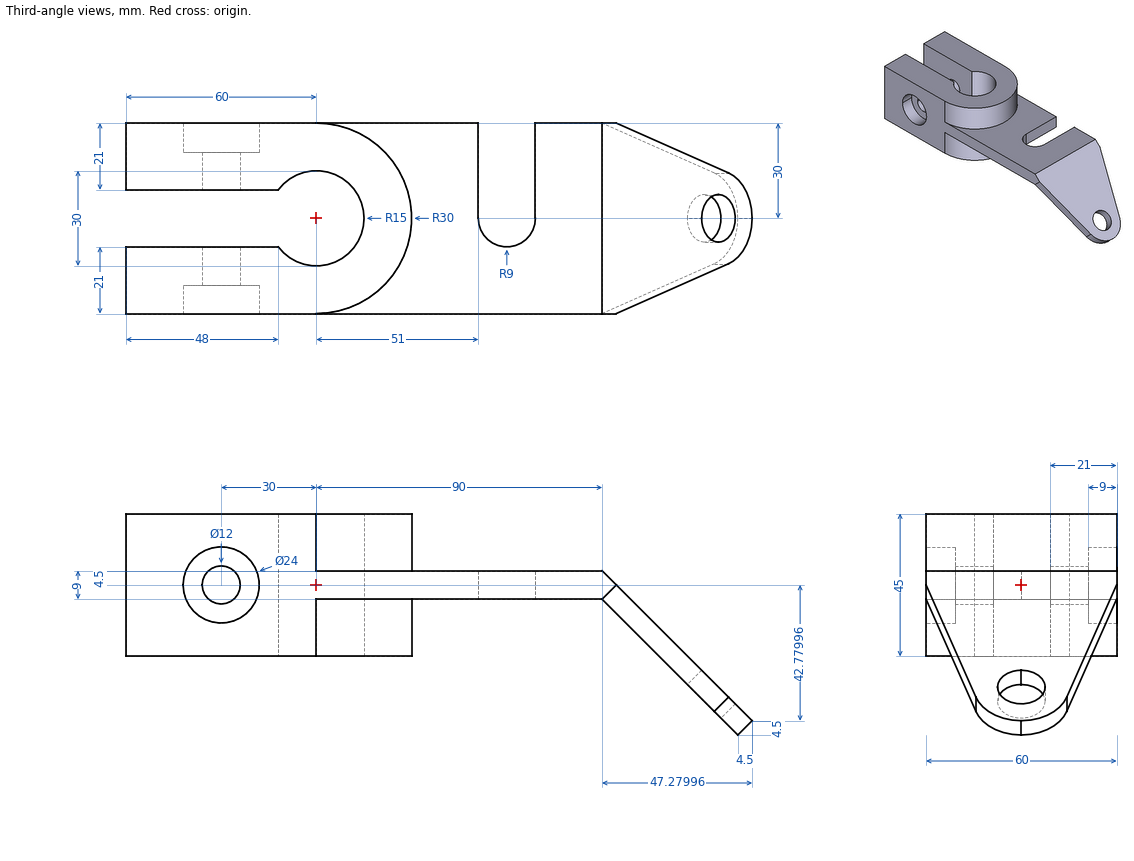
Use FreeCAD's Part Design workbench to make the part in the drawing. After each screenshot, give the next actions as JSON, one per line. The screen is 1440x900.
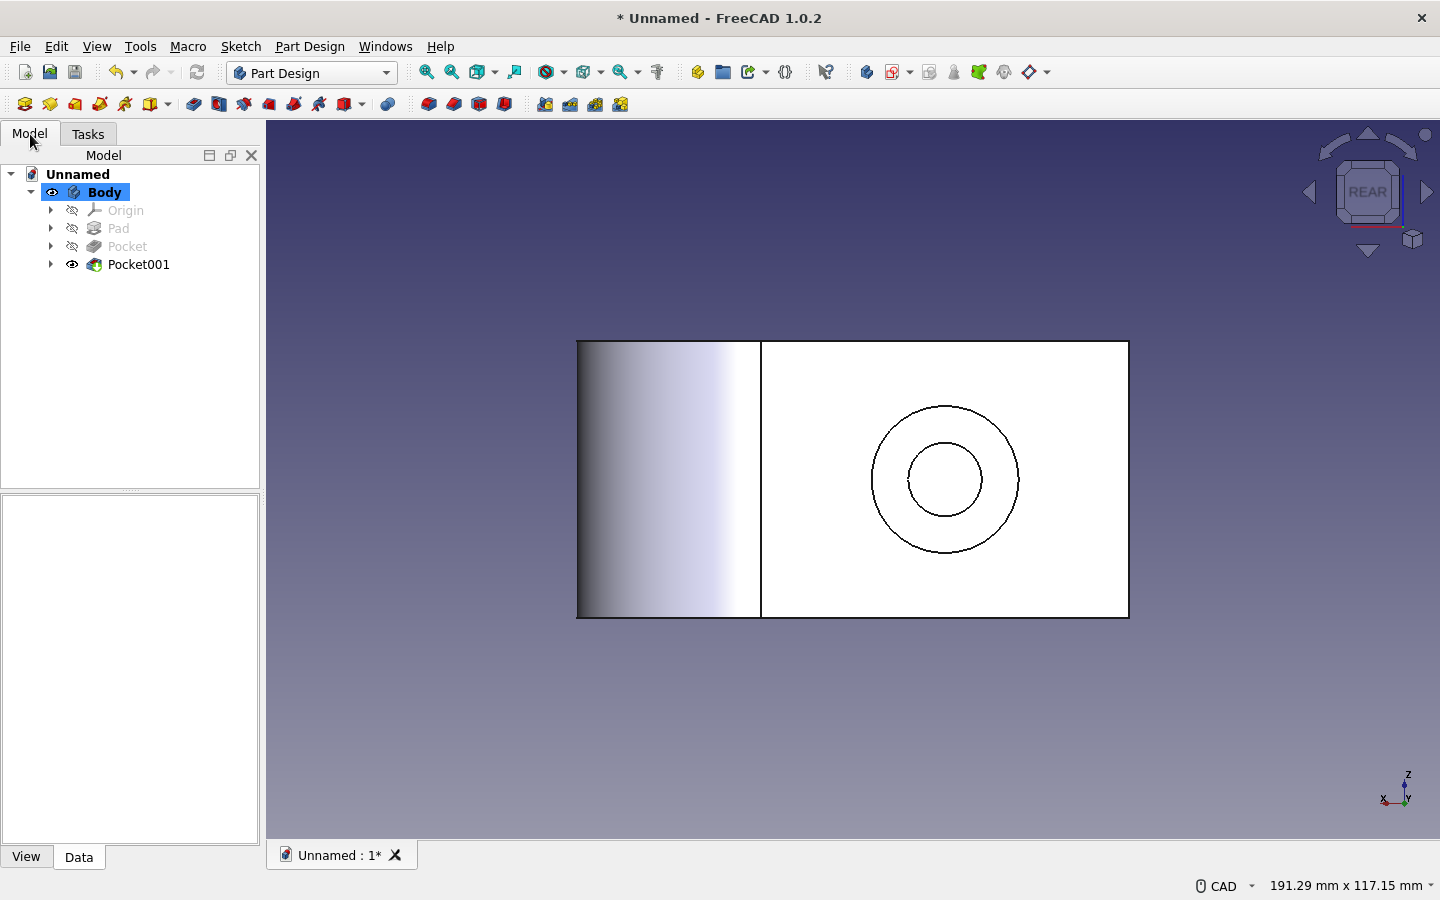
{"action": "left_click", "coordinate": [117, 246]}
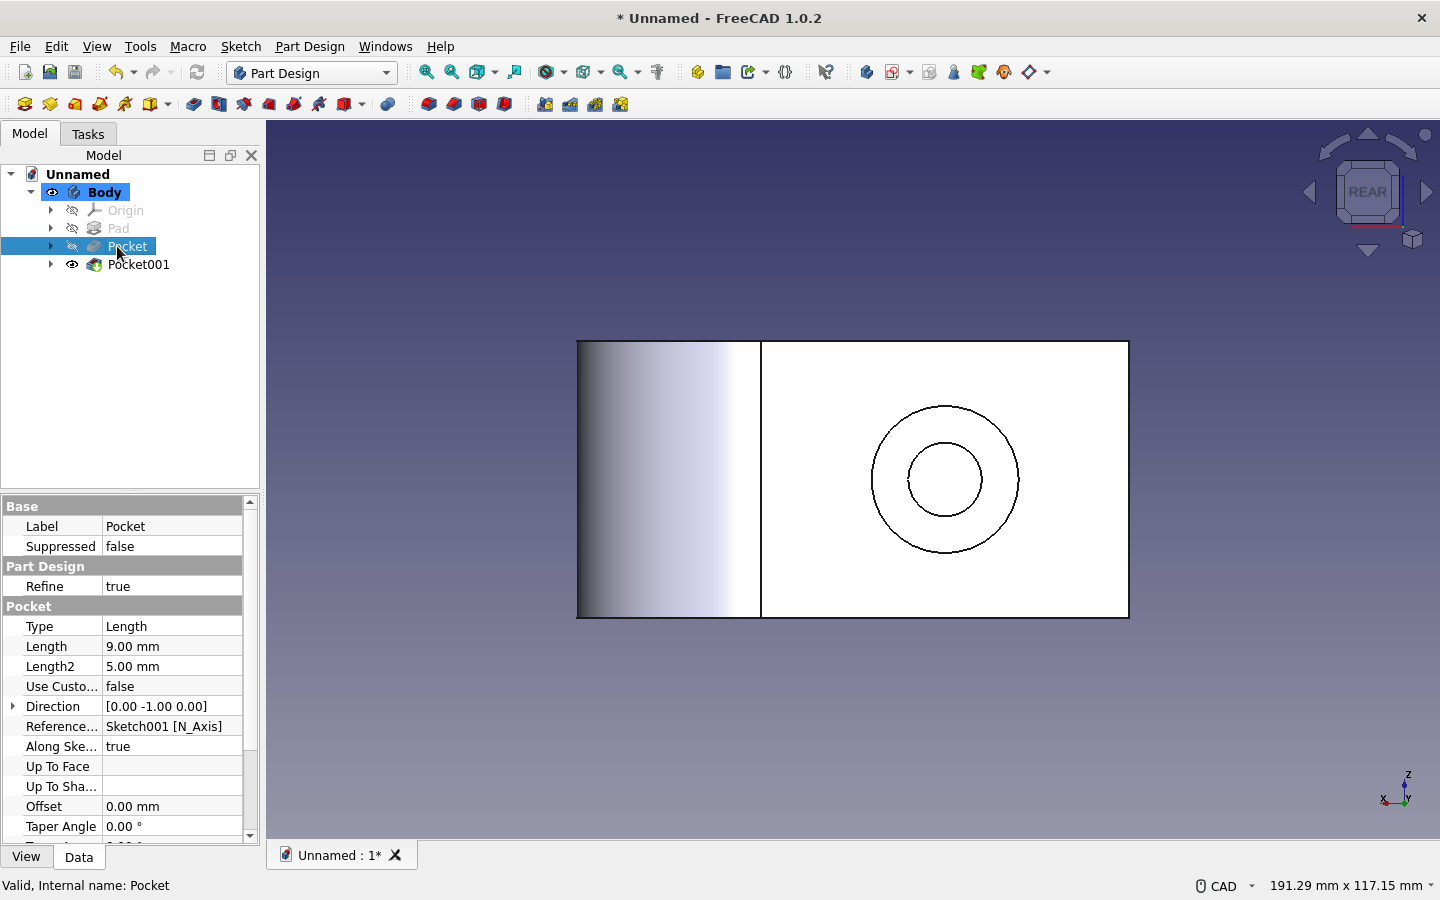
{"action": "left_click", "coordinate": [545, 104]}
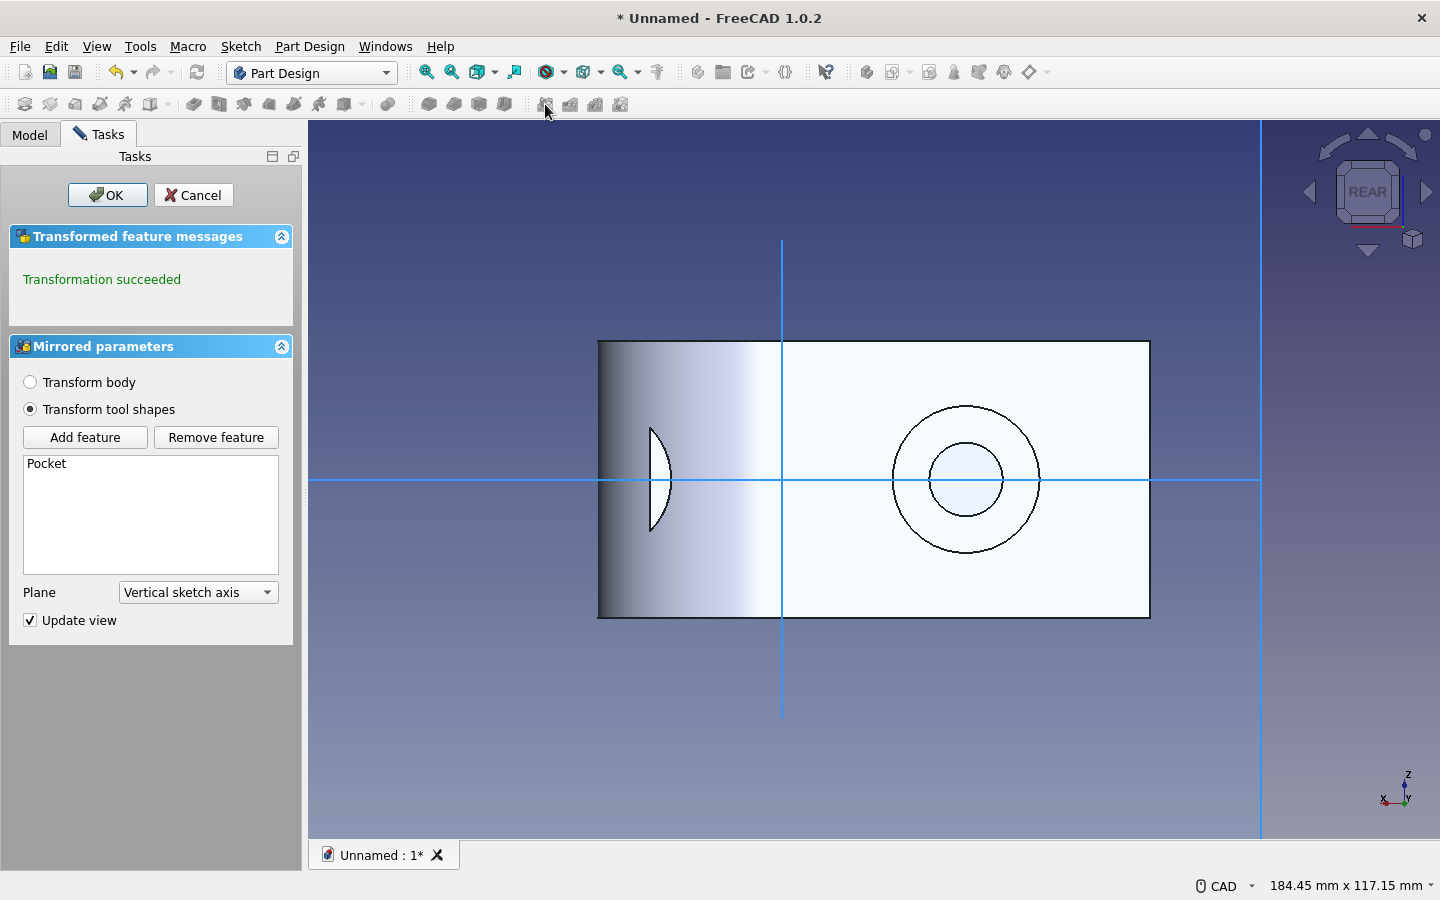
{"action": "left_click", "coordinate": [199, 592]}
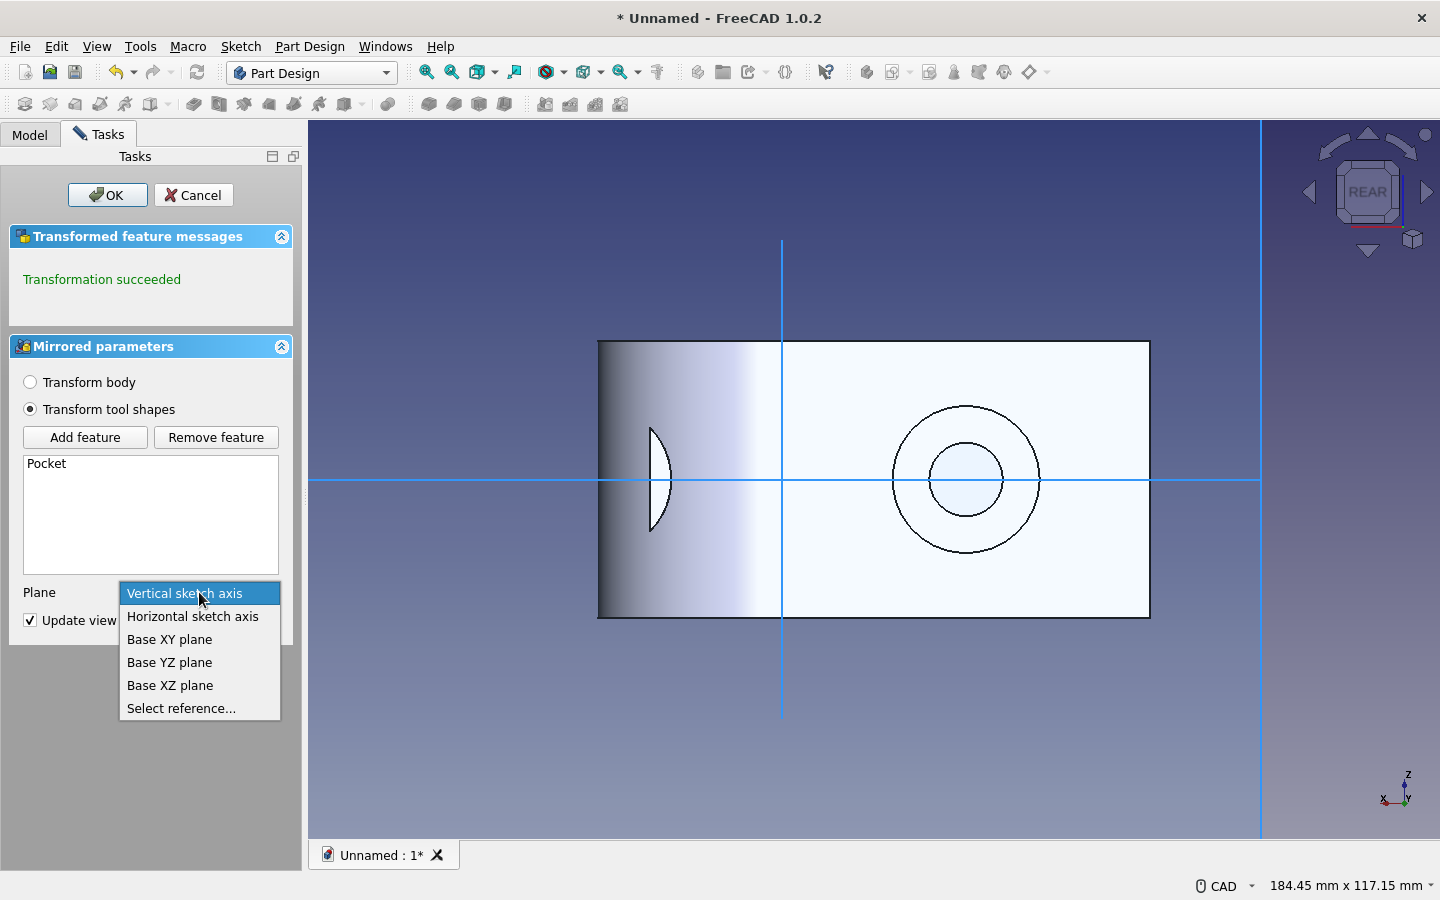
{"action": "left_click", "coordinate": [198, 686]}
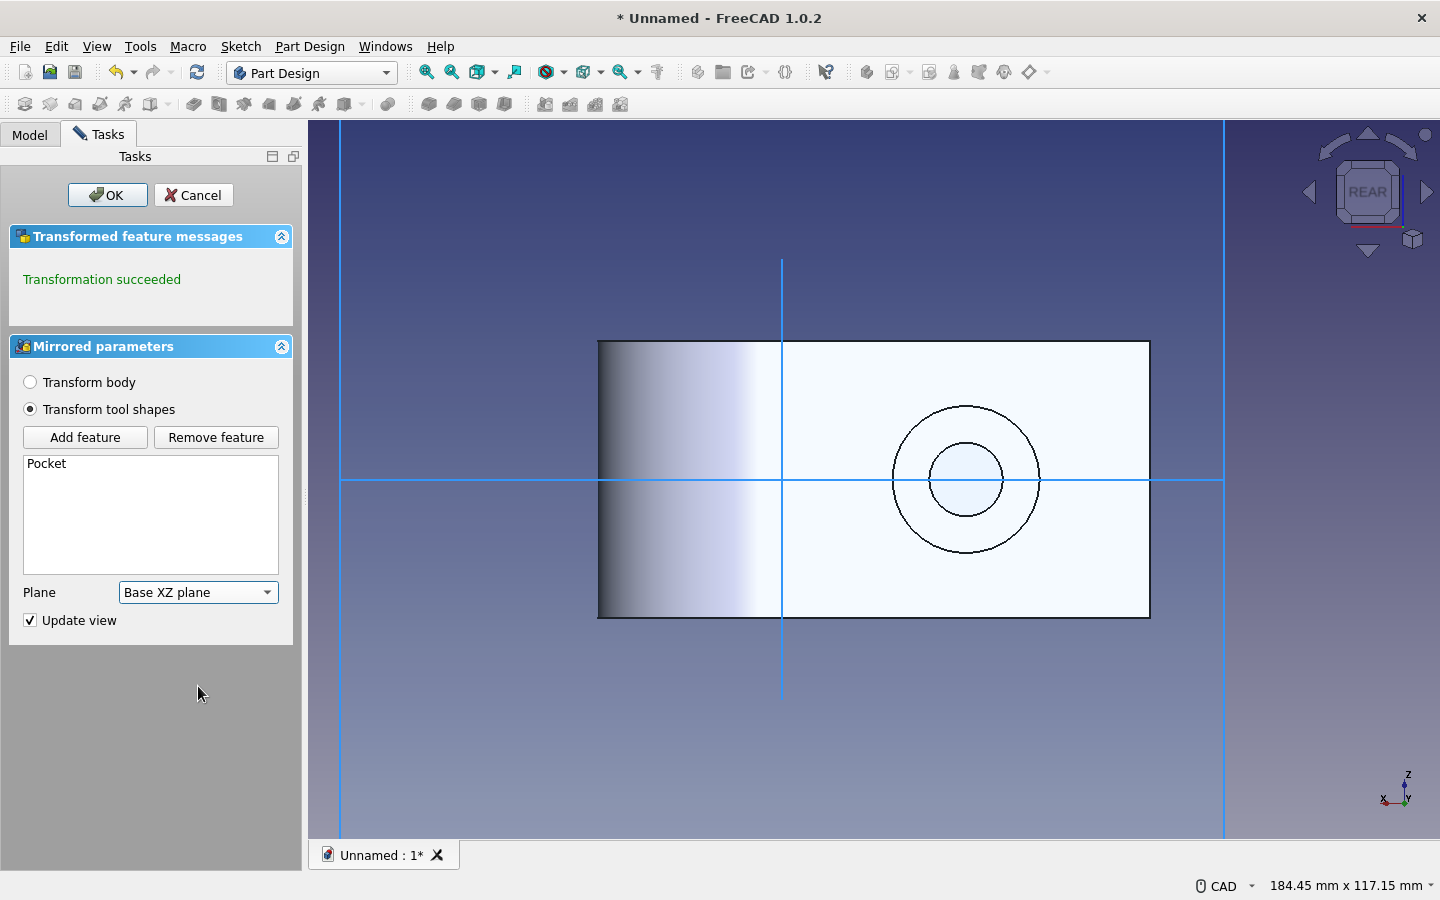
{"action": "left_click", "coordinate": [108, 195]}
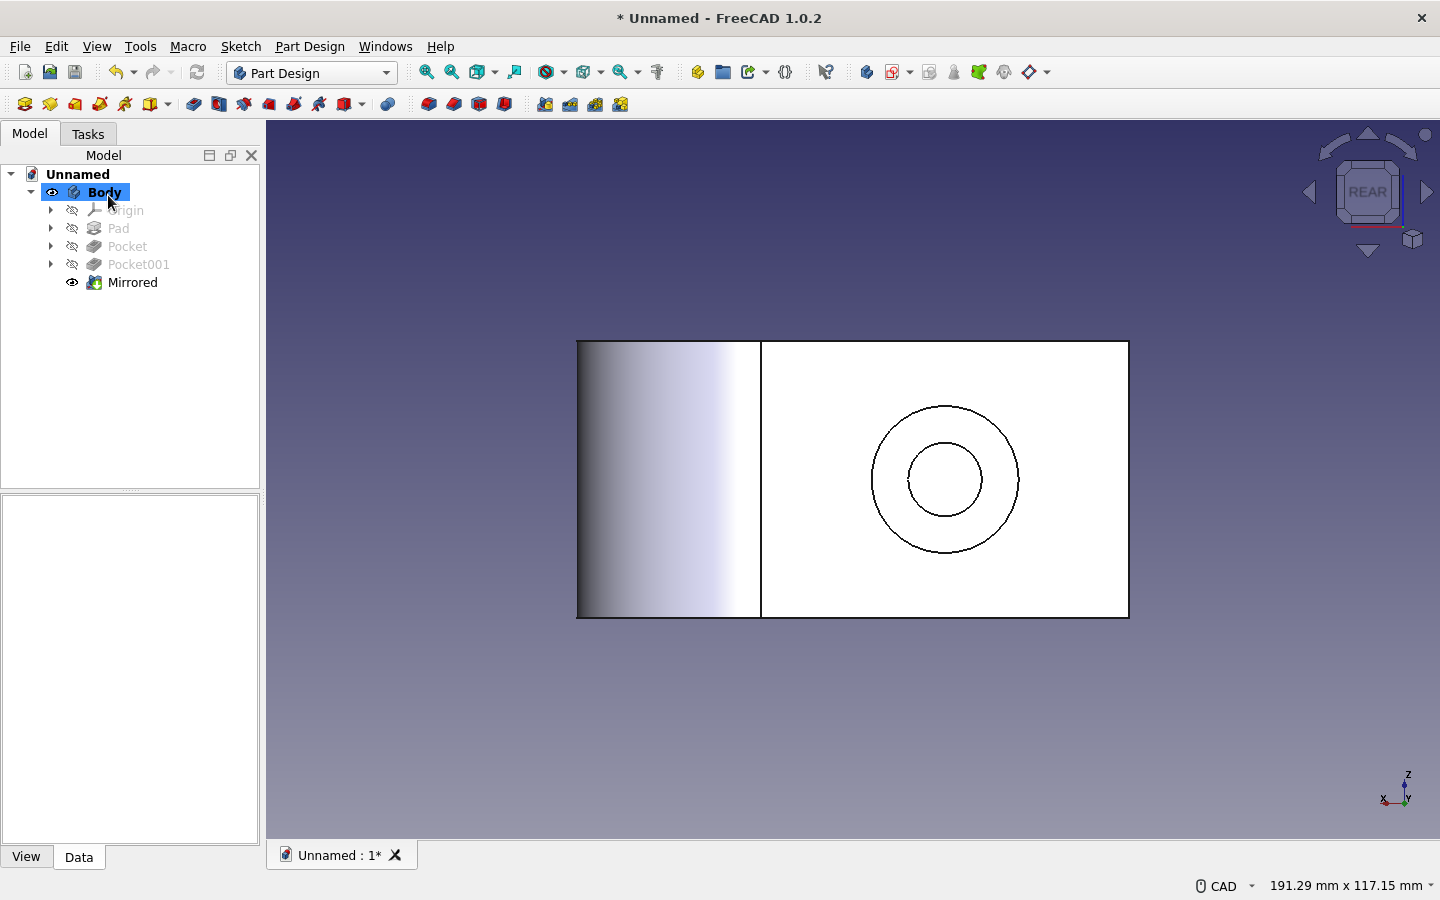
{"action": "left_click", "coordinate": [117, 264]}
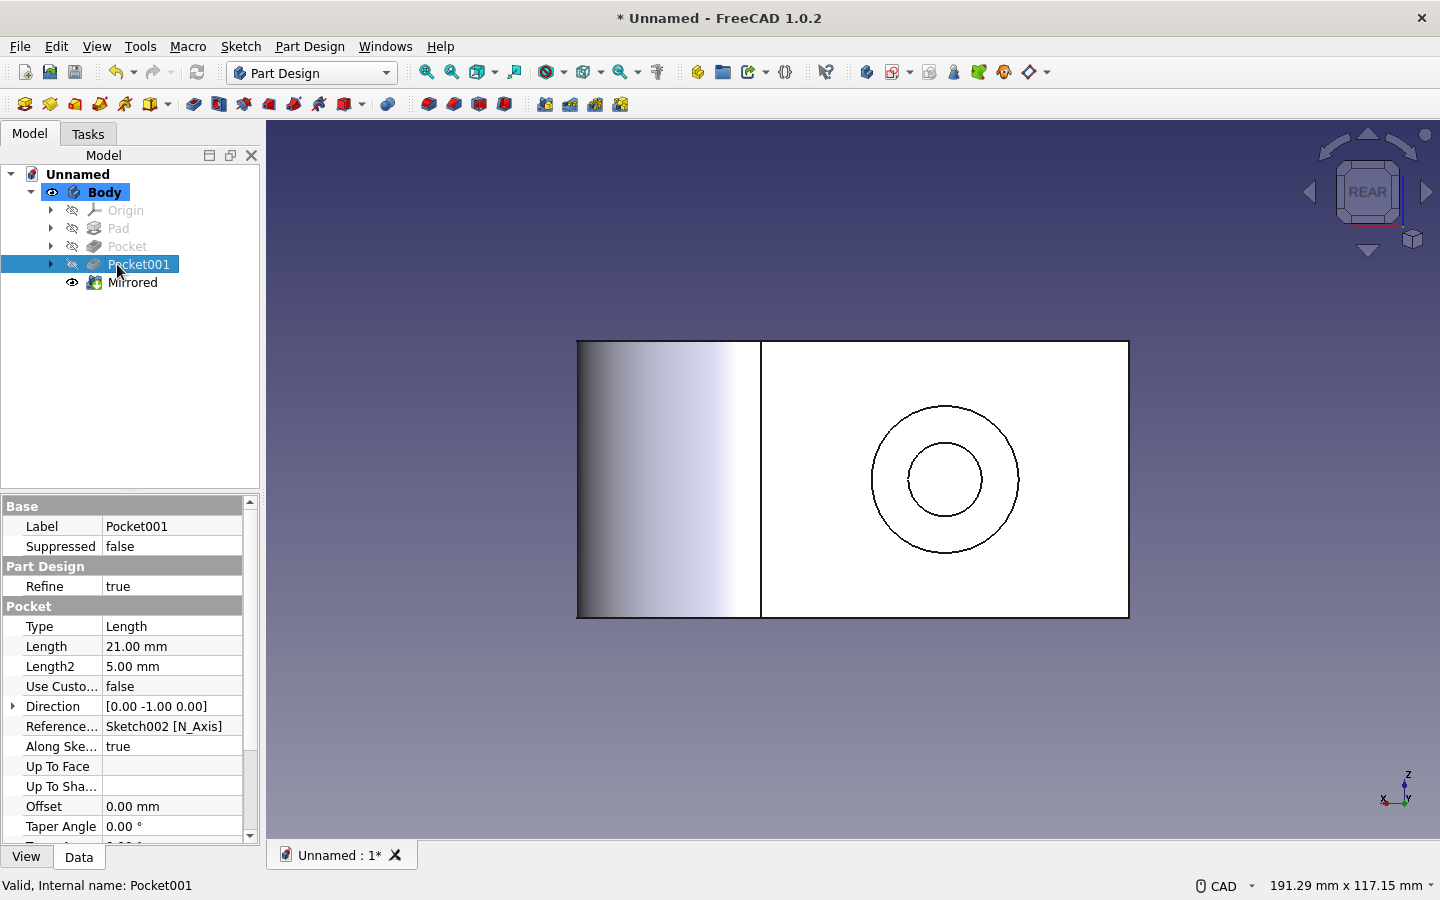
{"action": "left_click", "coordinate": [545, 104]}